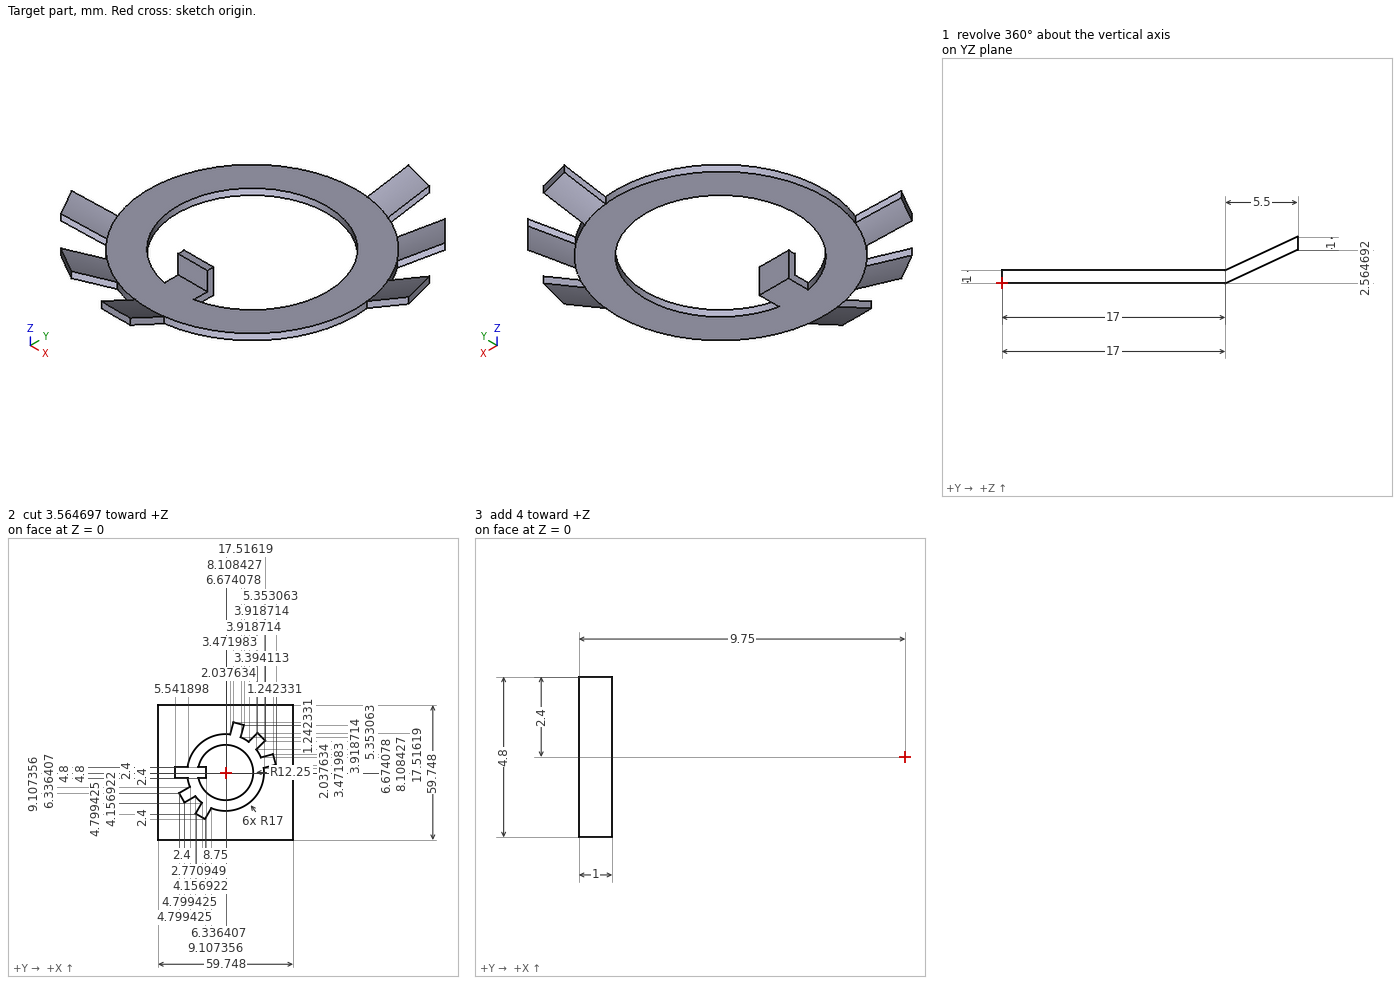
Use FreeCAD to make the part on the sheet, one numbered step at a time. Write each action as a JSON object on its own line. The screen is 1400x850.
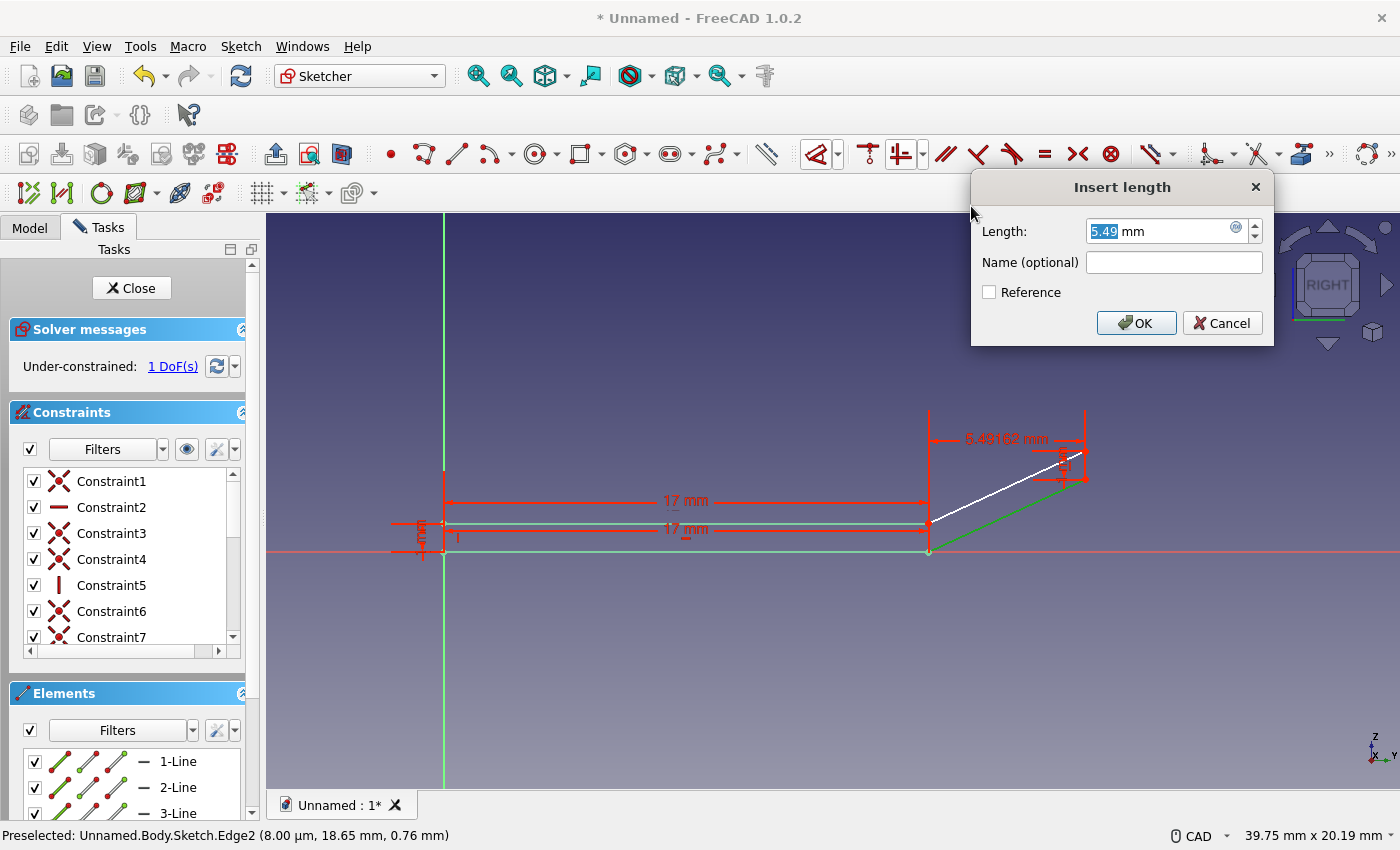
{"action": "type", "text": "5.5"}
{"action": "key", "text": "Return"}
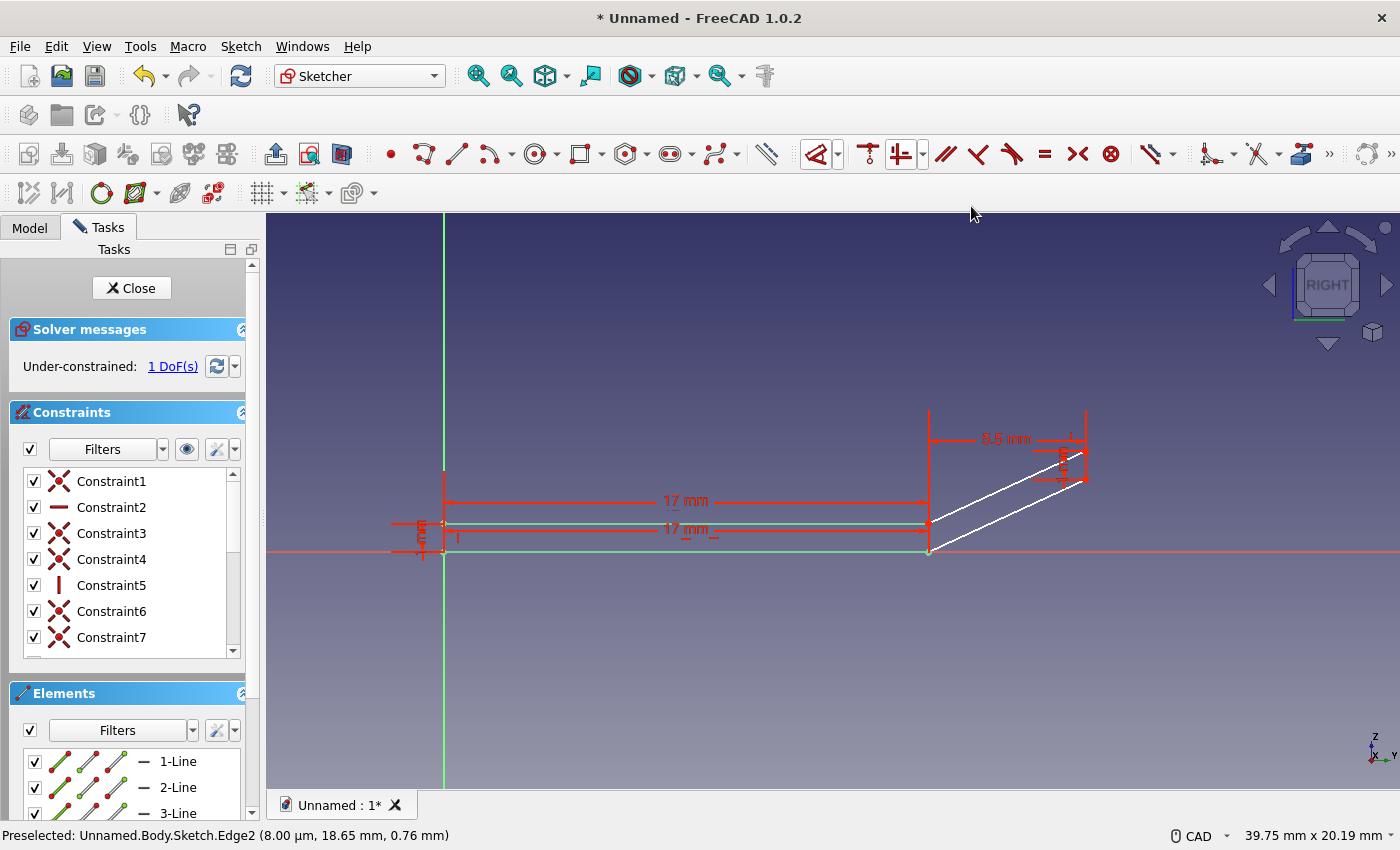
{"action": "left_click", "coordinate": [1086, 480]}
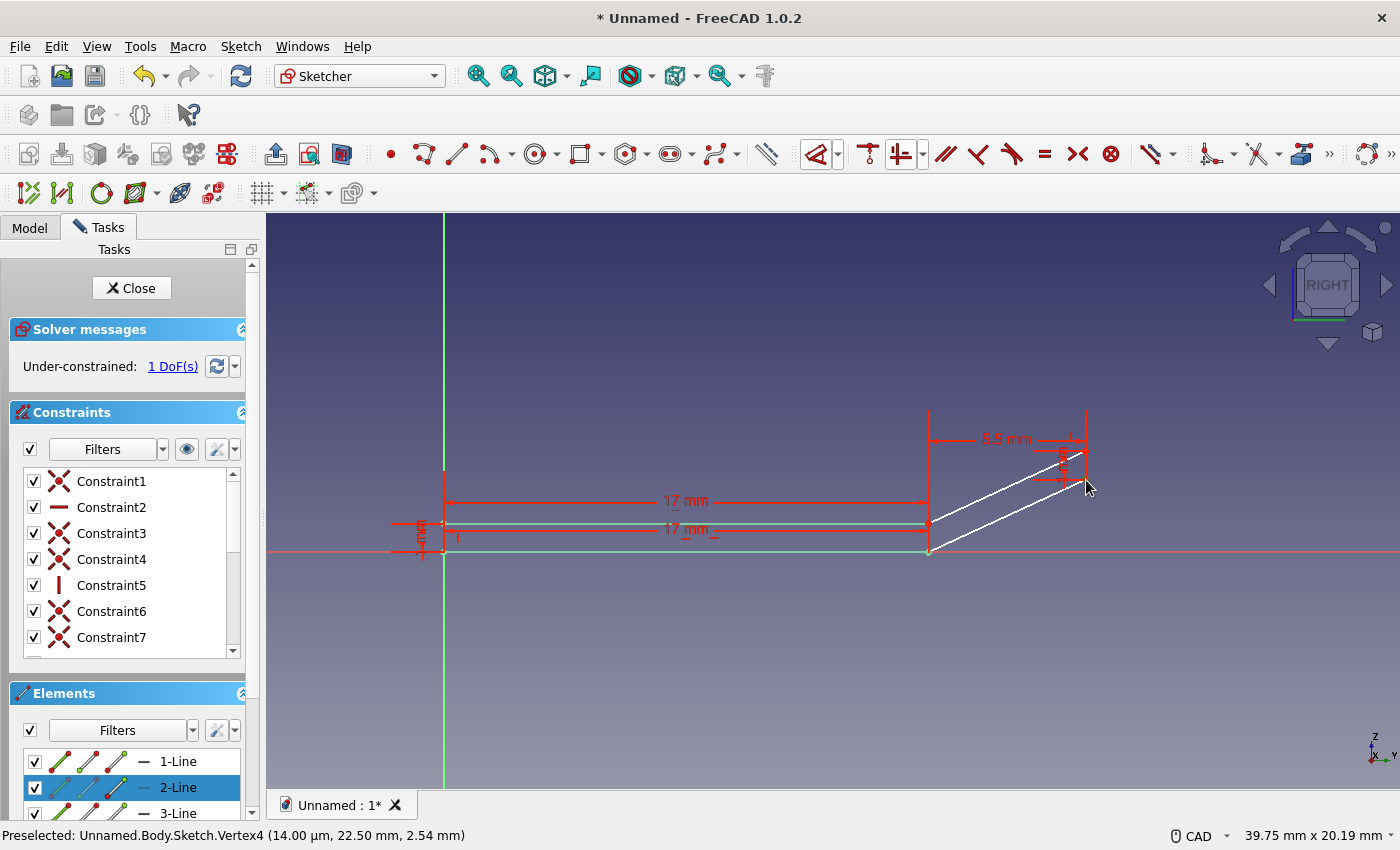
{"action": "key", "text": "i"}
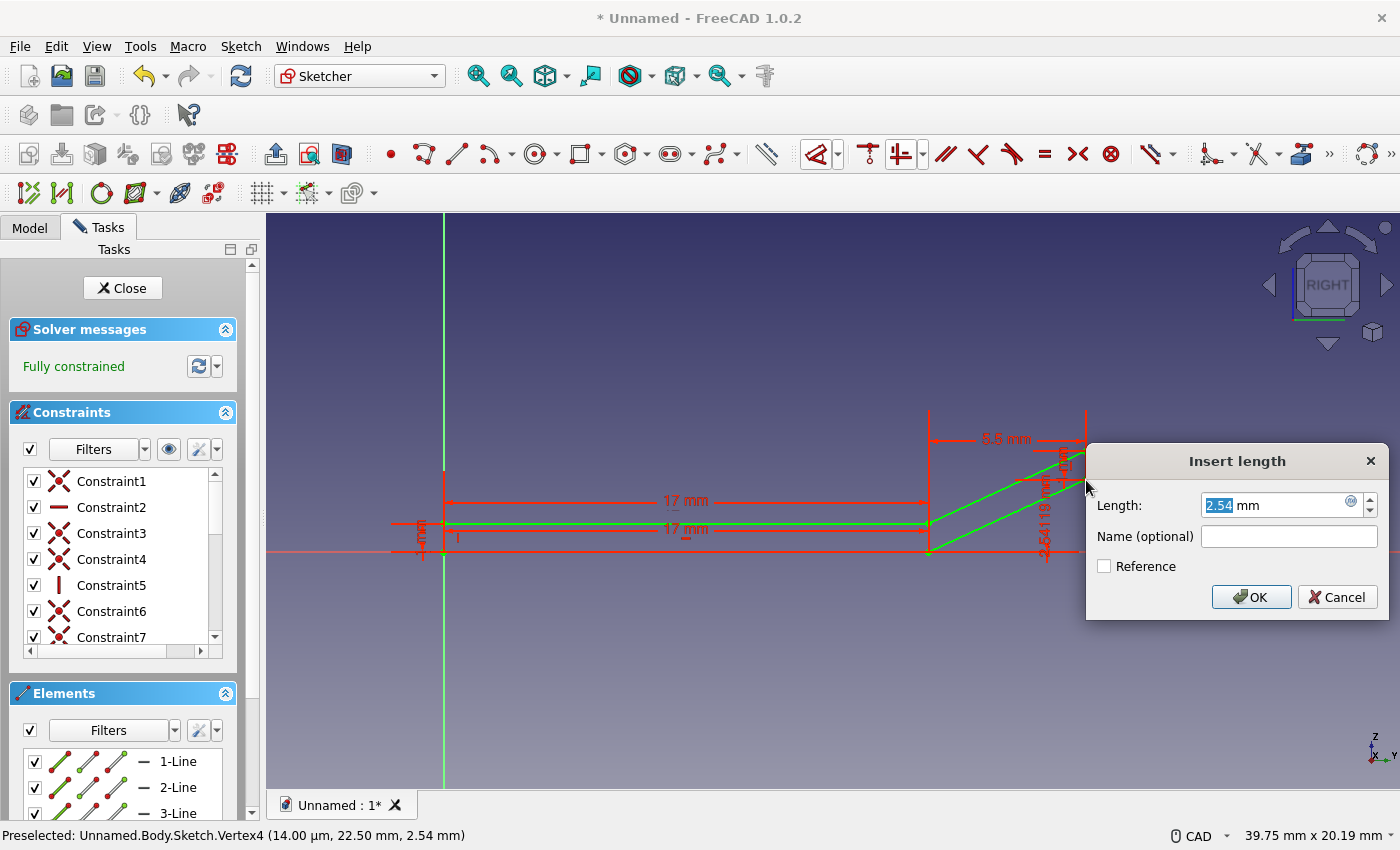
{"action": "type", "text": "2.564692"}
{"action": "key", "text": "Return"}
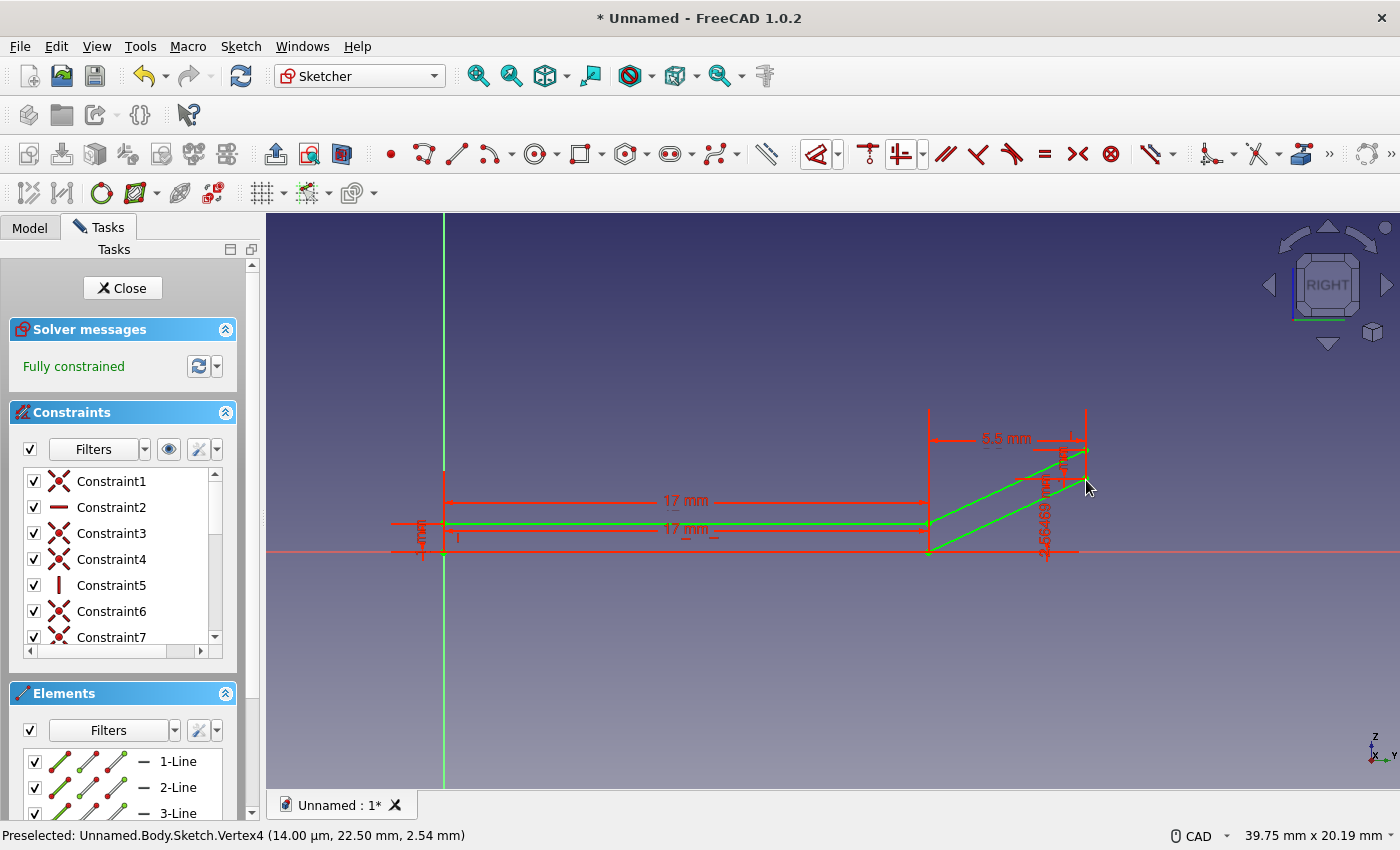
{"action": "left_click", "coordinate": [123, 288]}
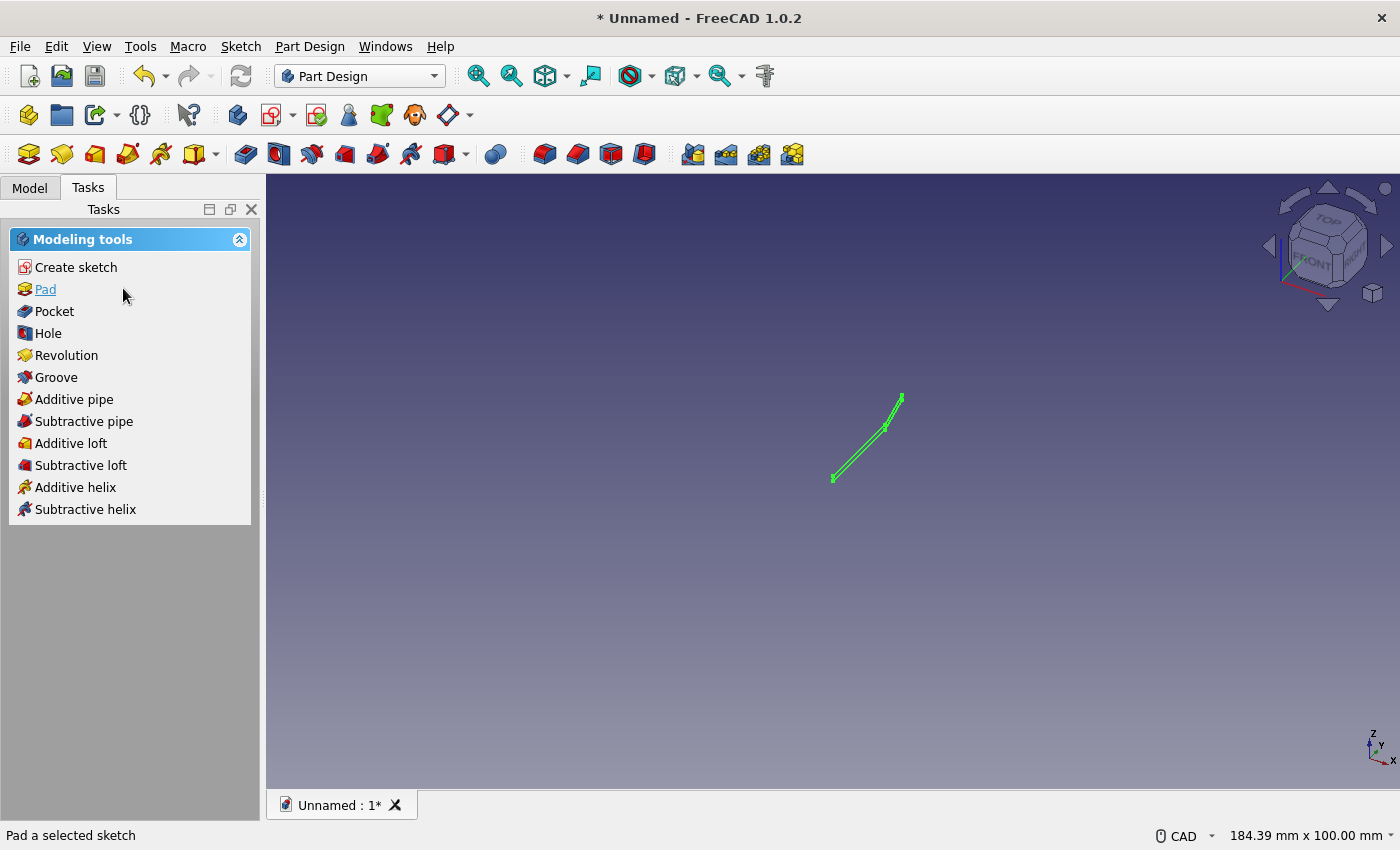
{"action": "left_click", "coordinate": [62, 154]}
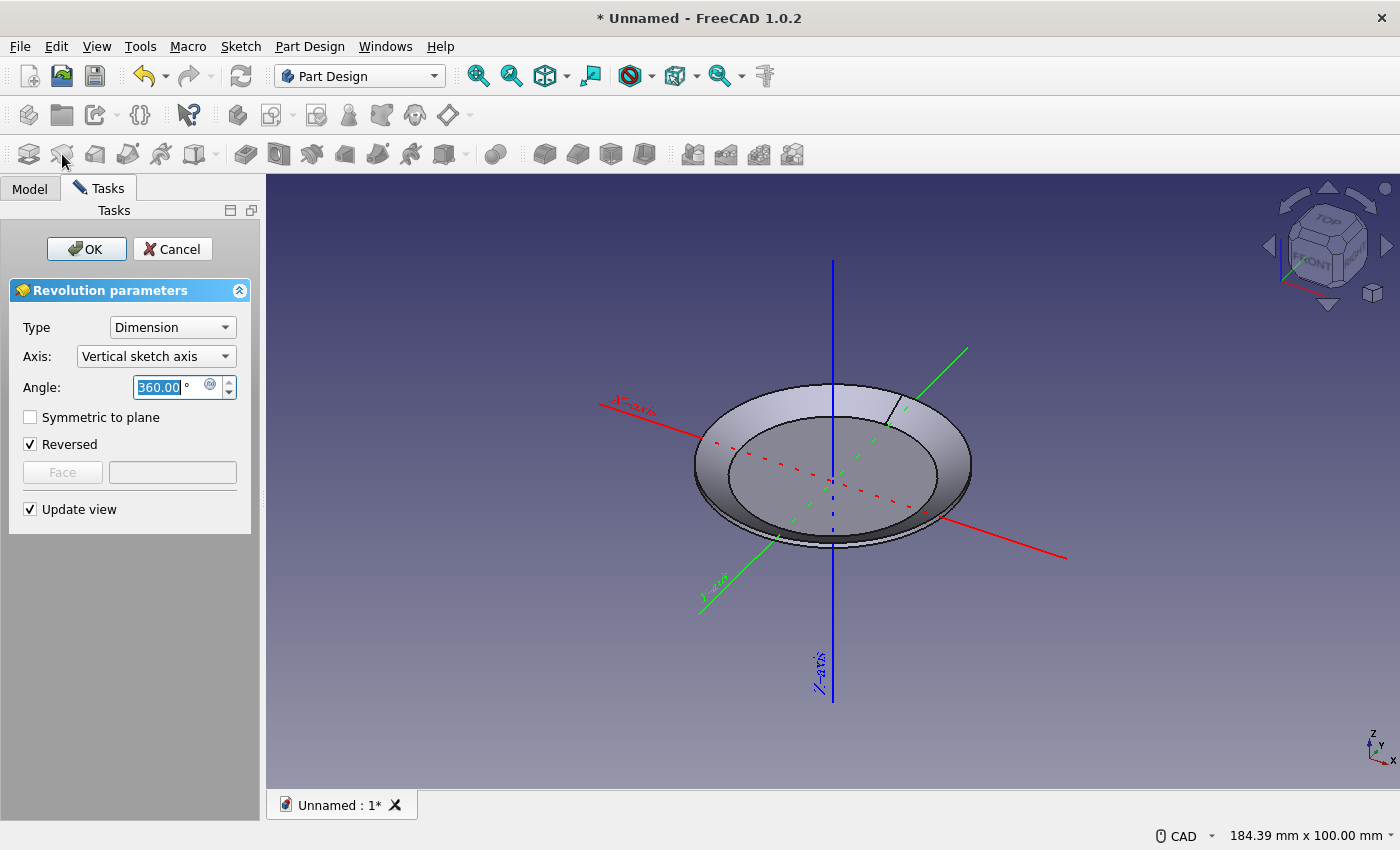
{"action": "left_click", "coordinate": [87, 249]}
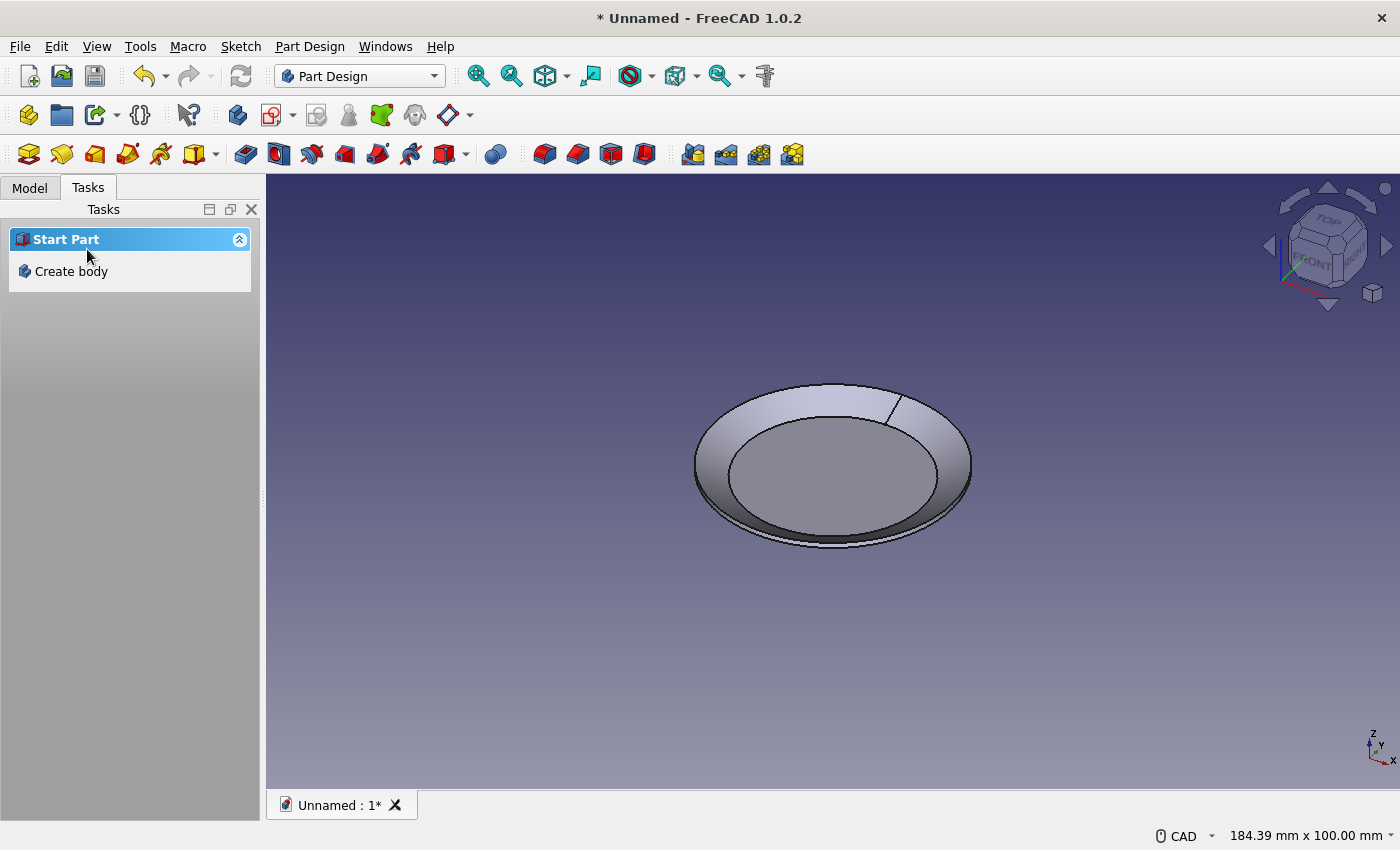
{"action": "left_click", "coordinate": [479, 76]}